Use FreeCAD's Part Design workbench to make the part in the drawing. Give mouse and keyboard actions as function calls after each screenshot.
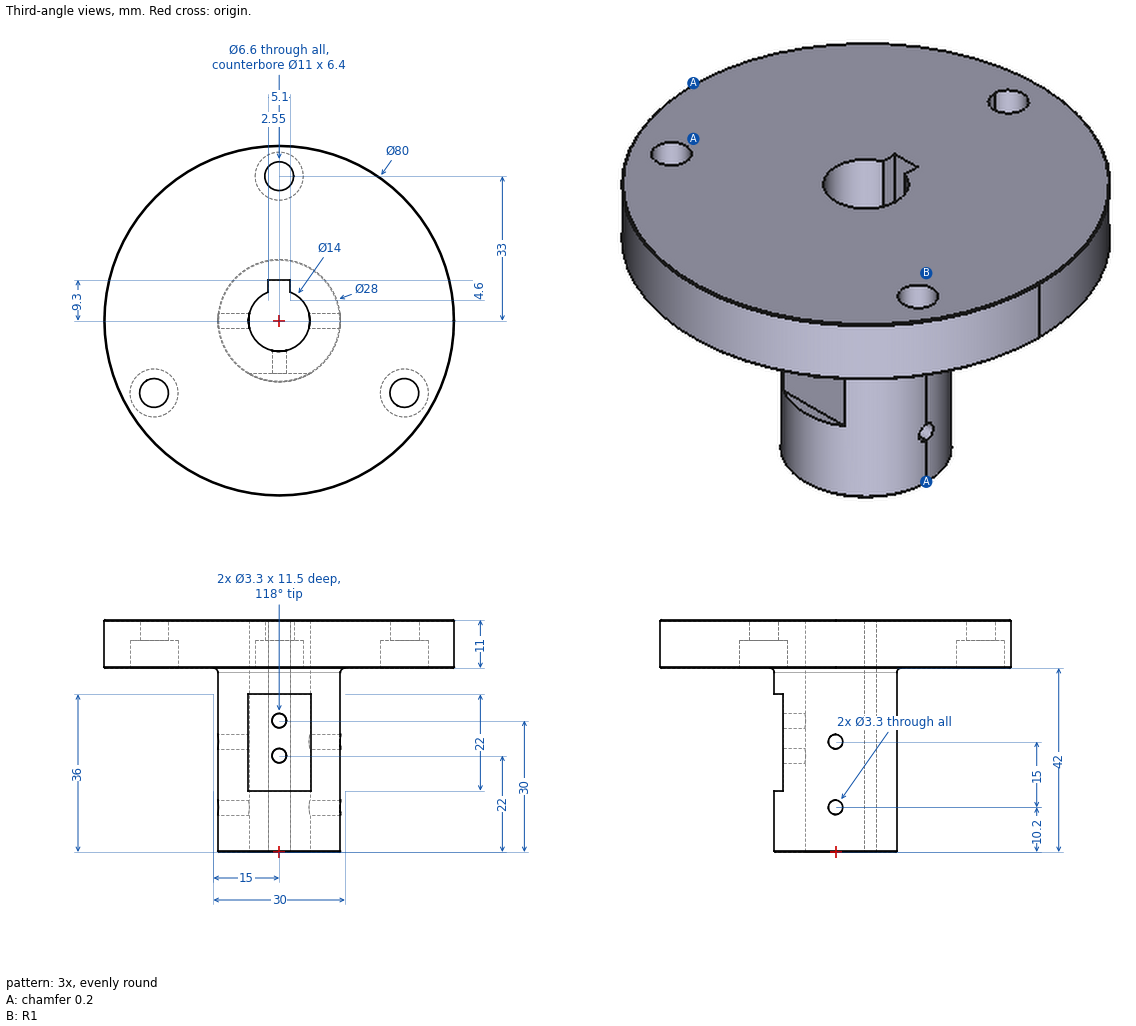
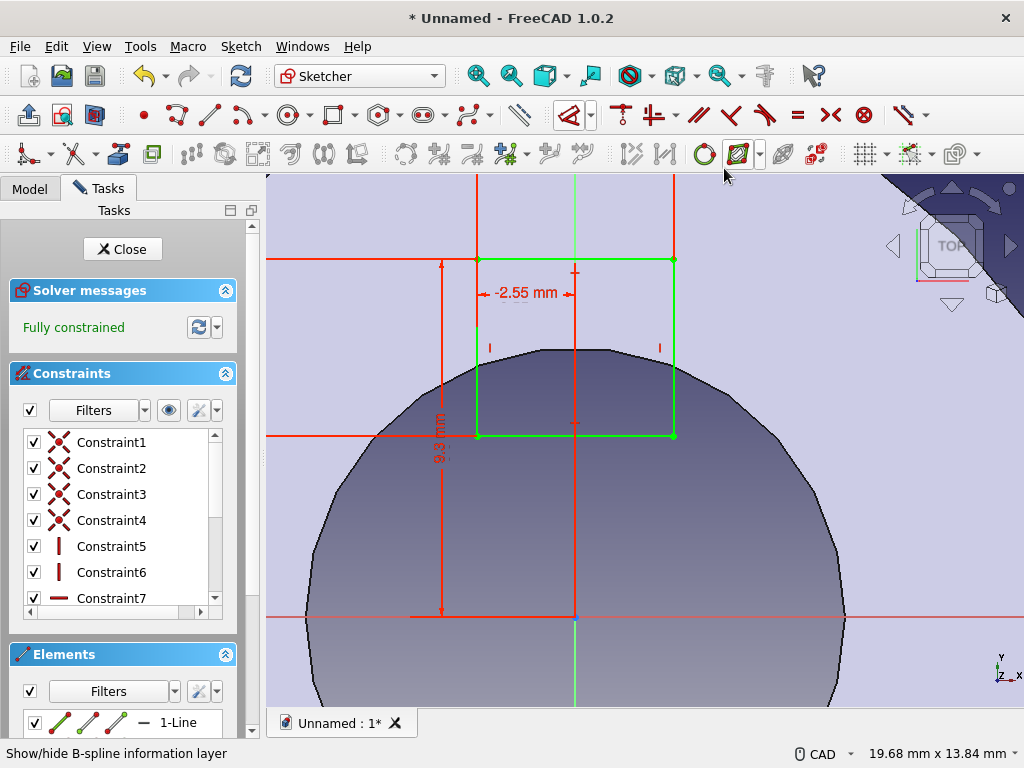
click(123, 249)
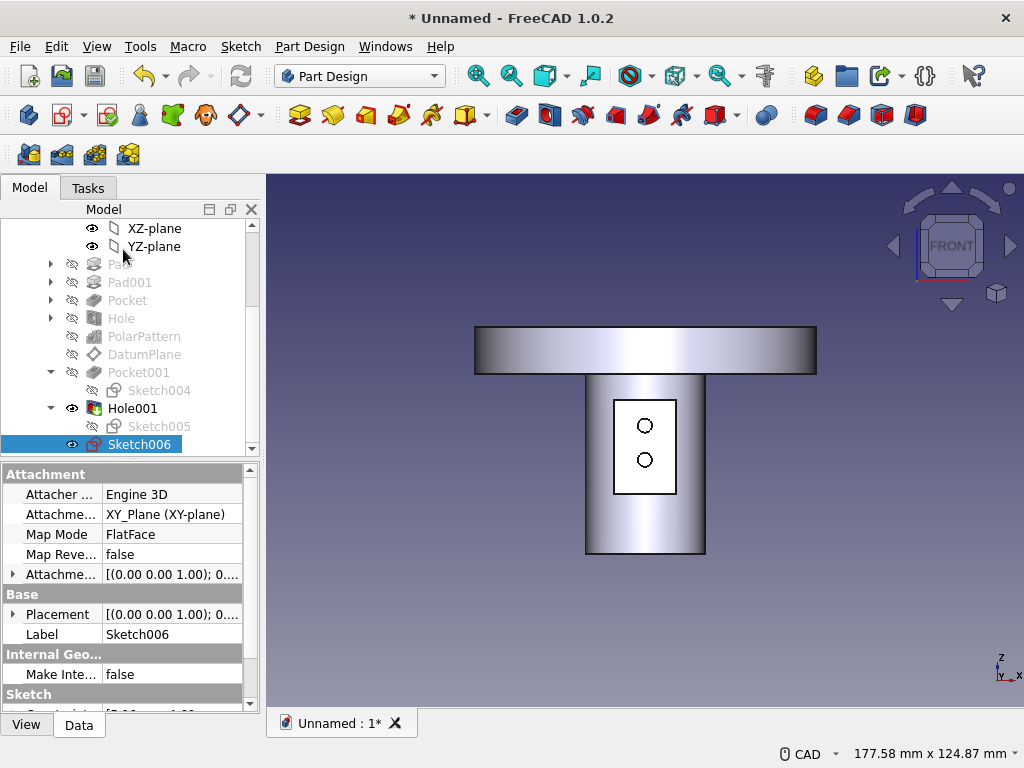
click(517, 116)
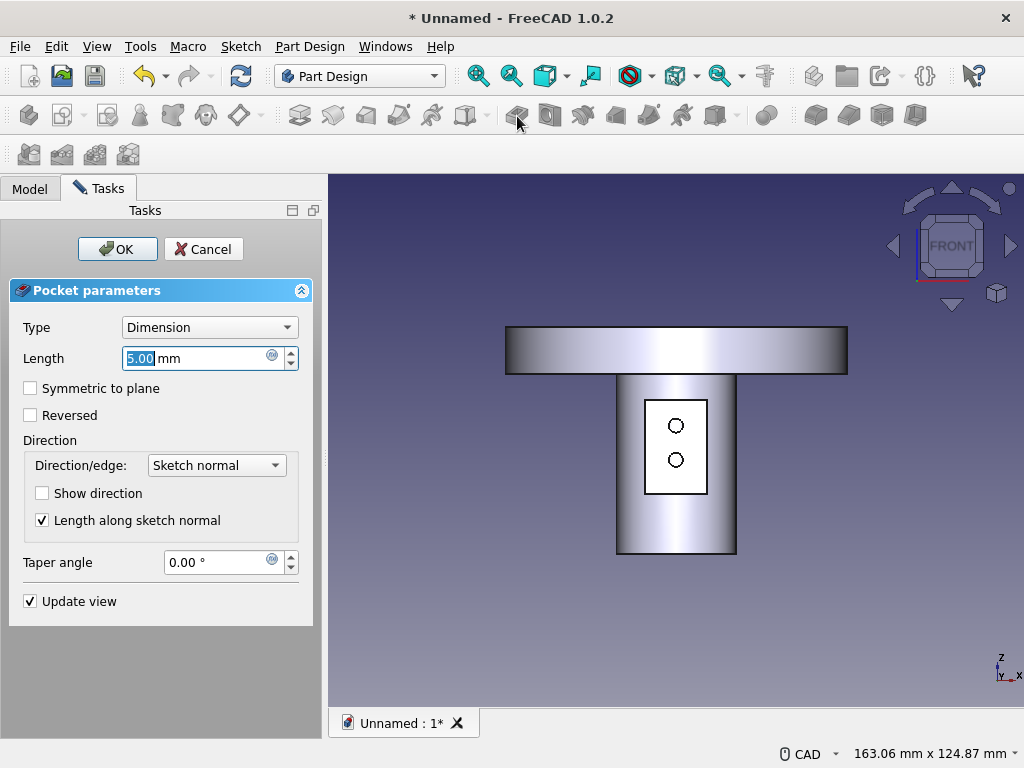
click(210, 328)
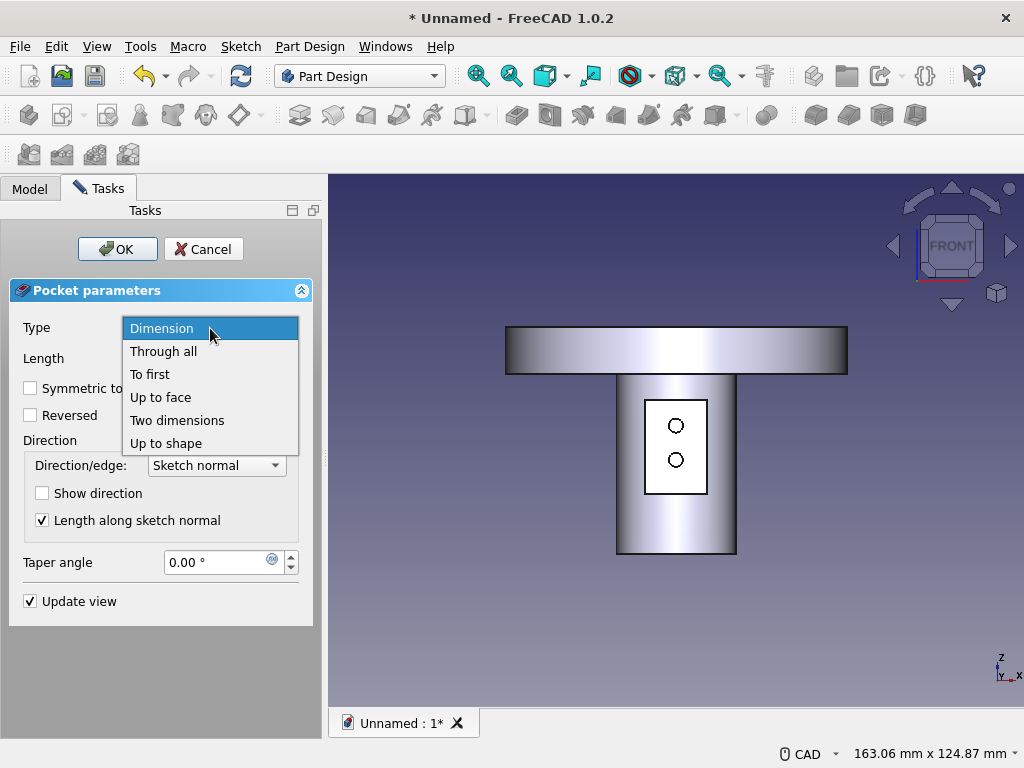
click(208, 352)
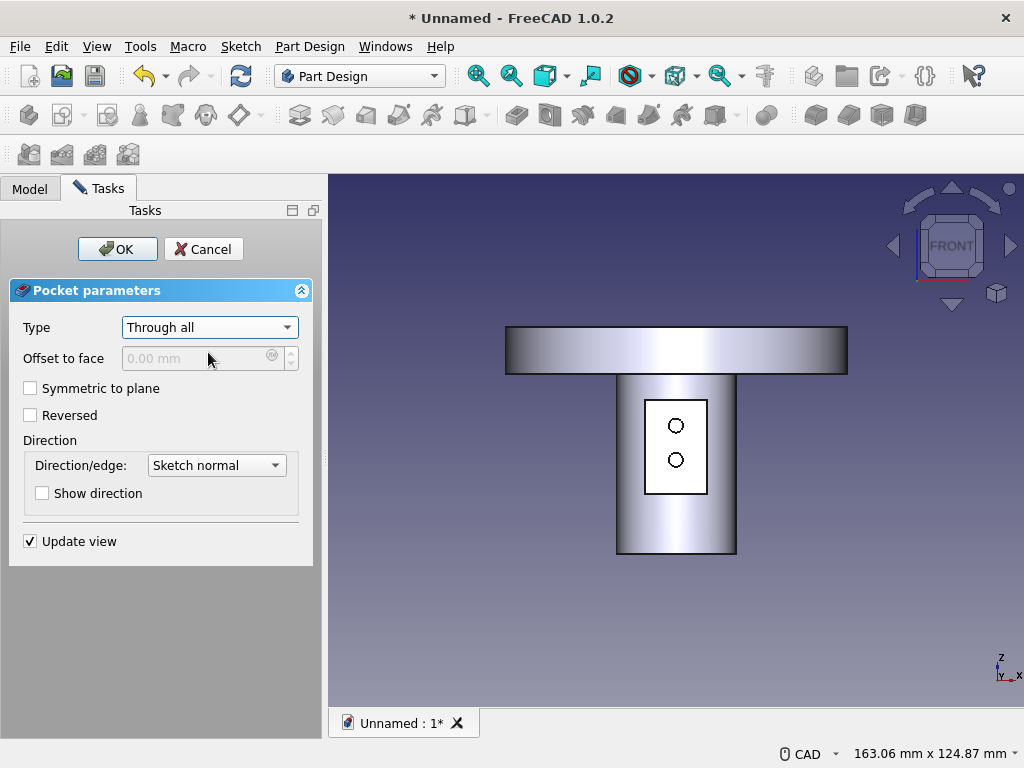
click(31, 415)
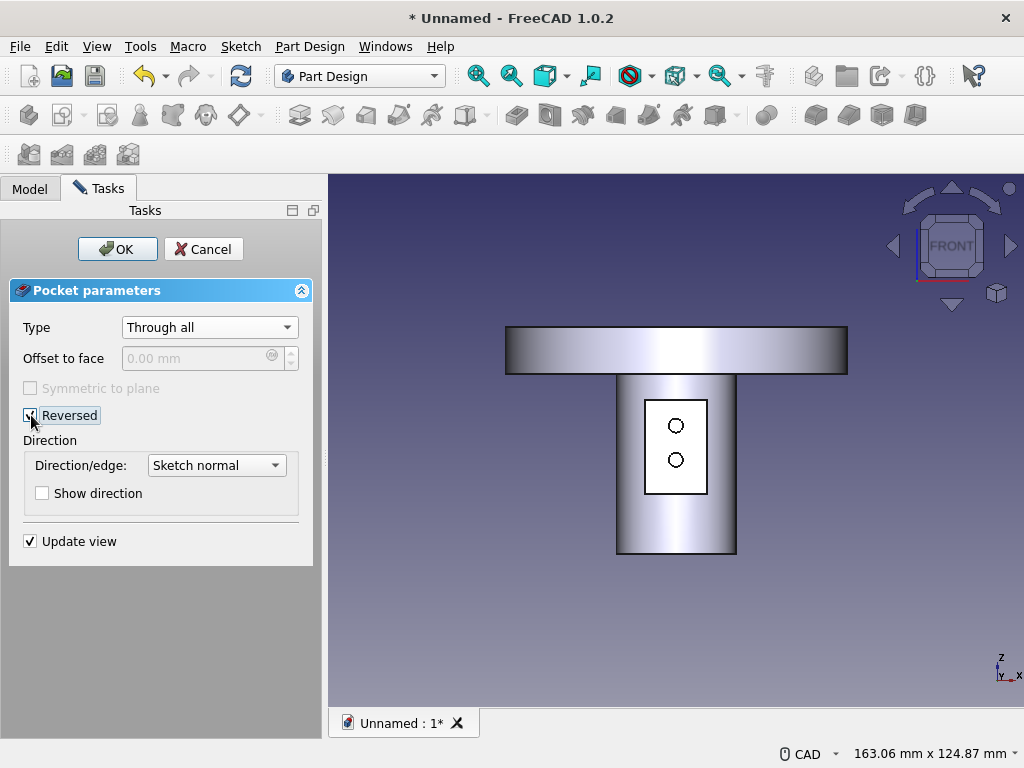
click(118, 249)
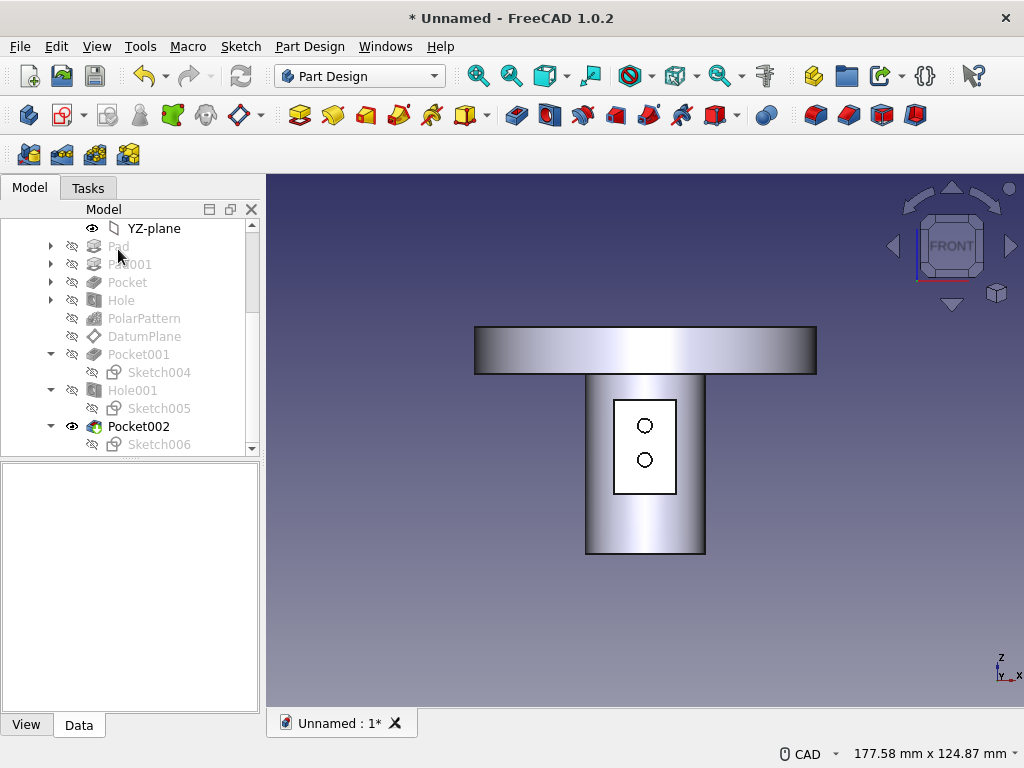
click(597, 553)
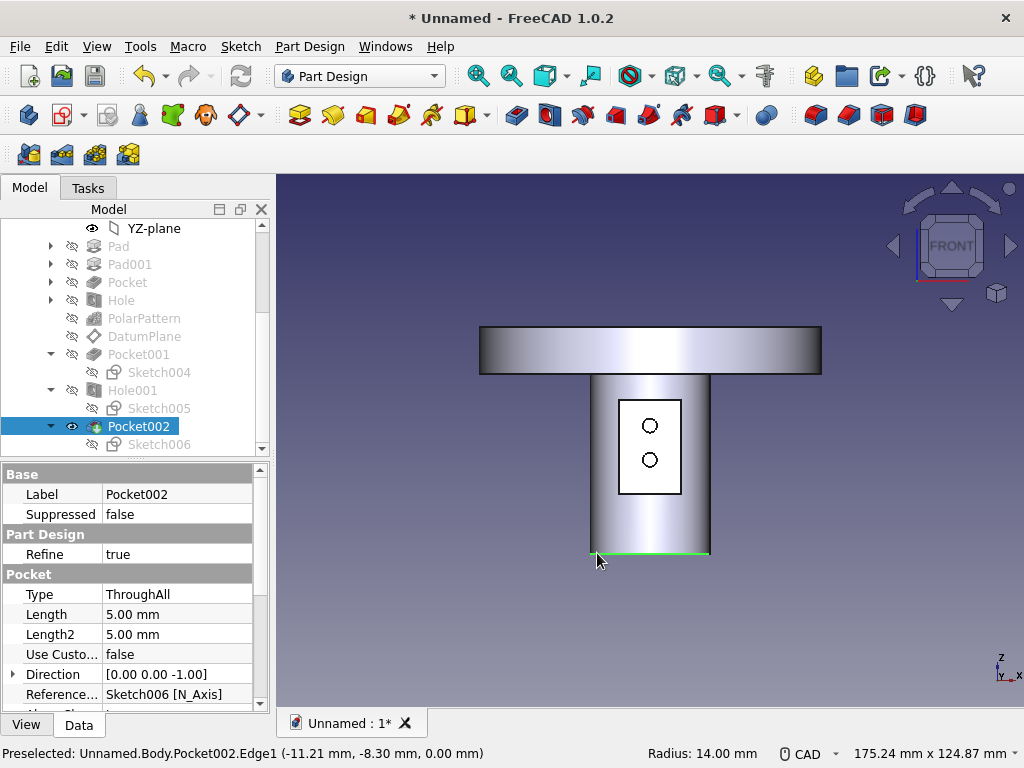
click(512, 373, ctrl)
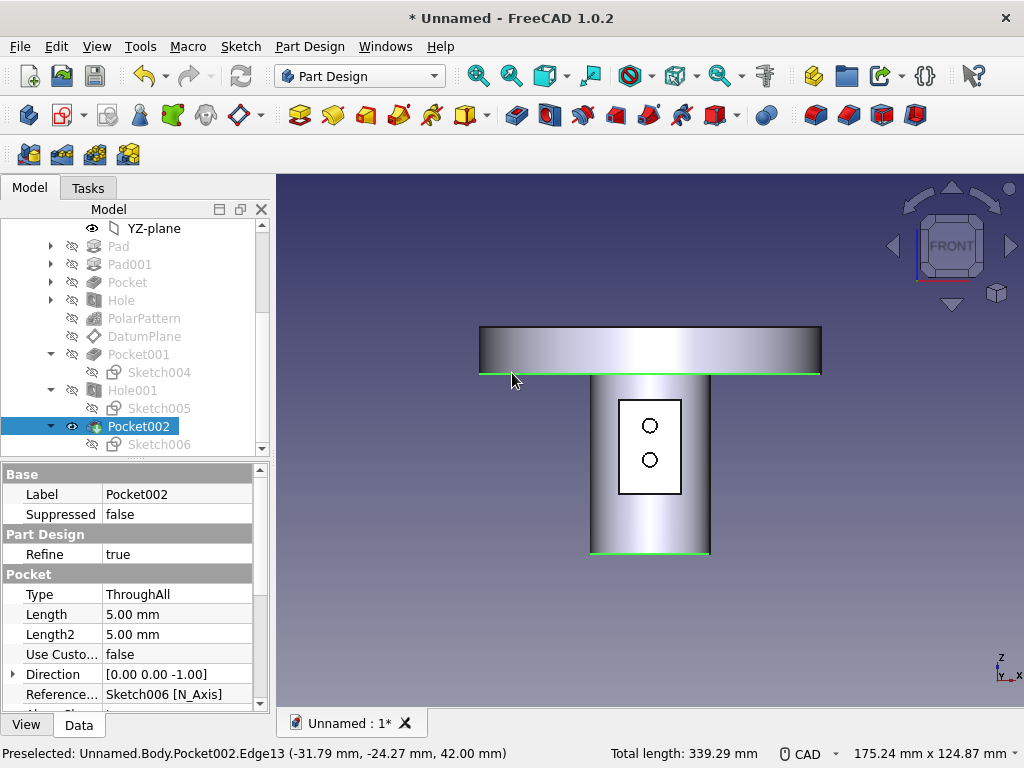
click(512, 326, ctrl)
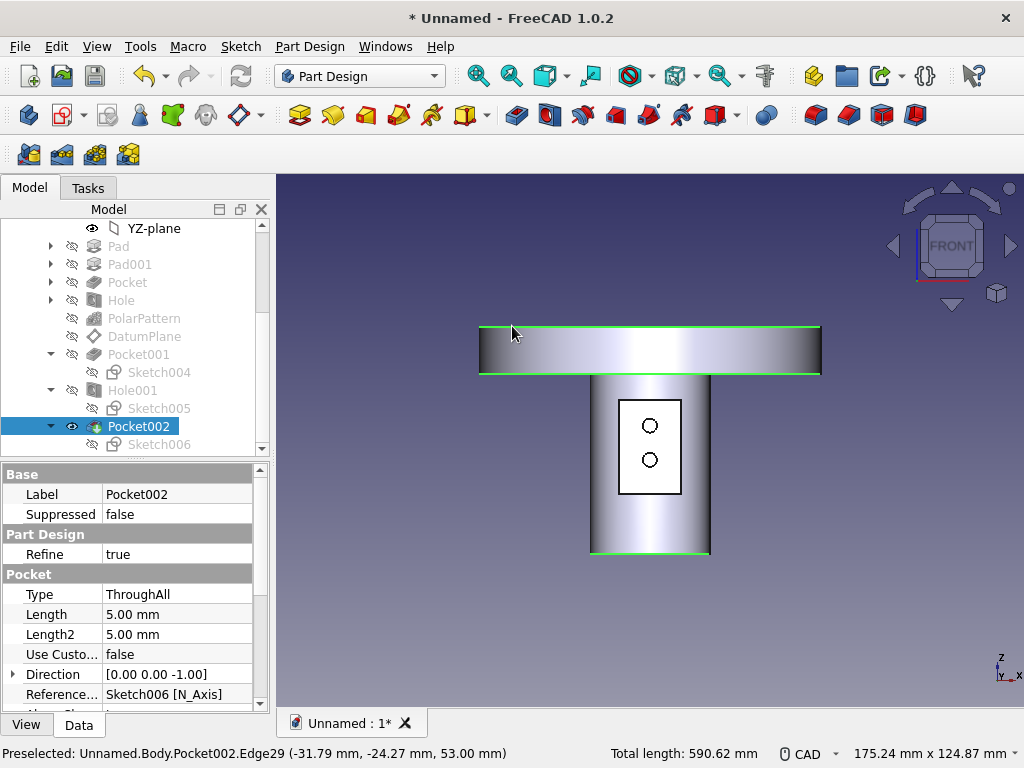
click(849, 116)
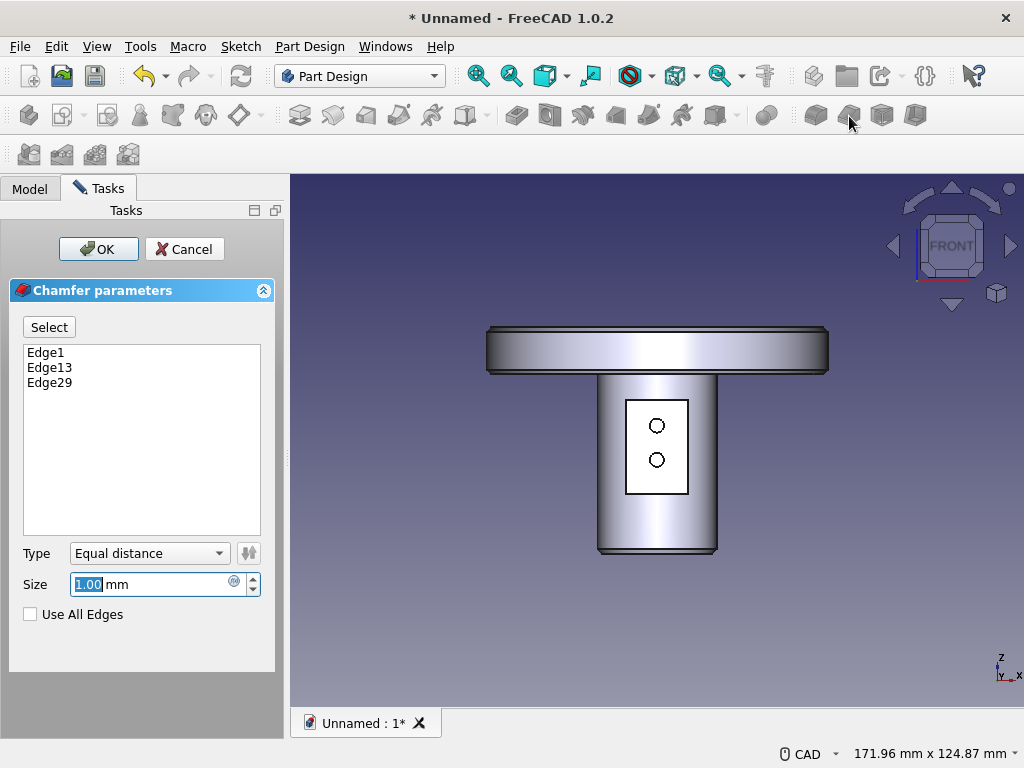
text(0.2)
key(Tab)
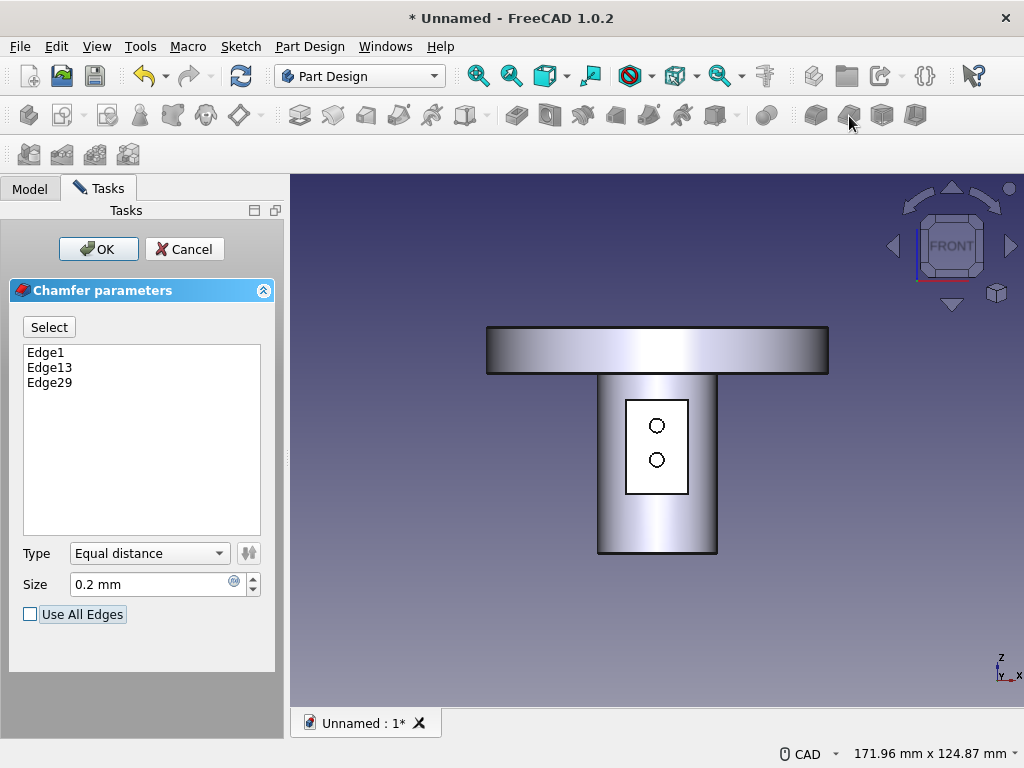
click(99, 249)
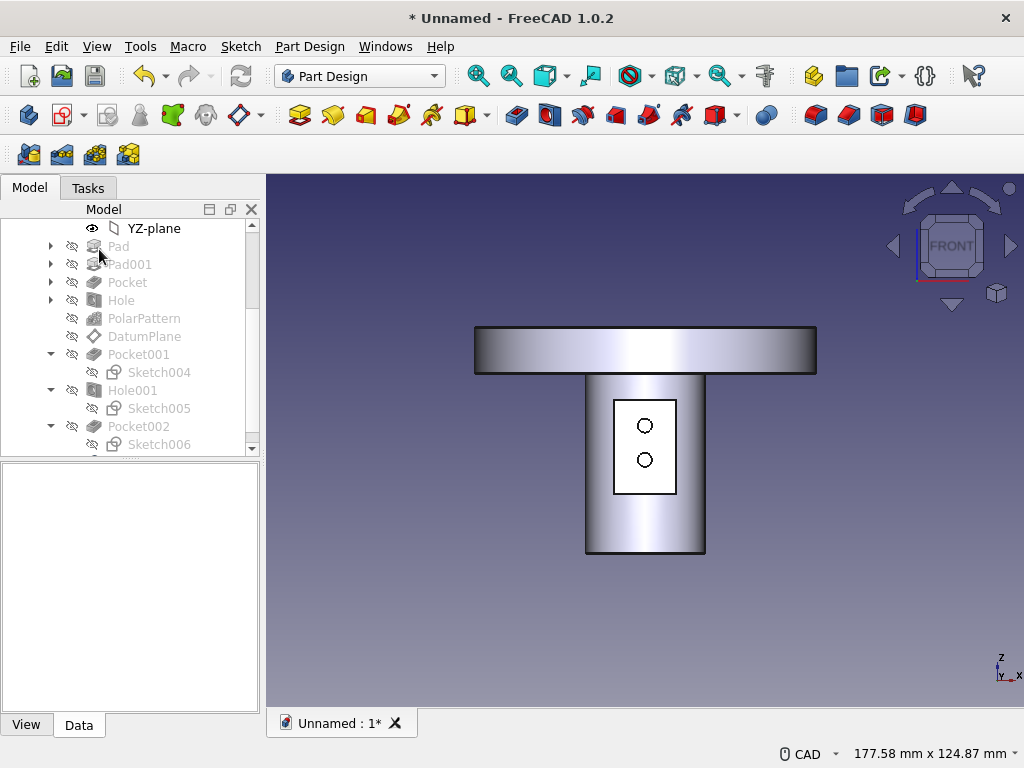
key(0)